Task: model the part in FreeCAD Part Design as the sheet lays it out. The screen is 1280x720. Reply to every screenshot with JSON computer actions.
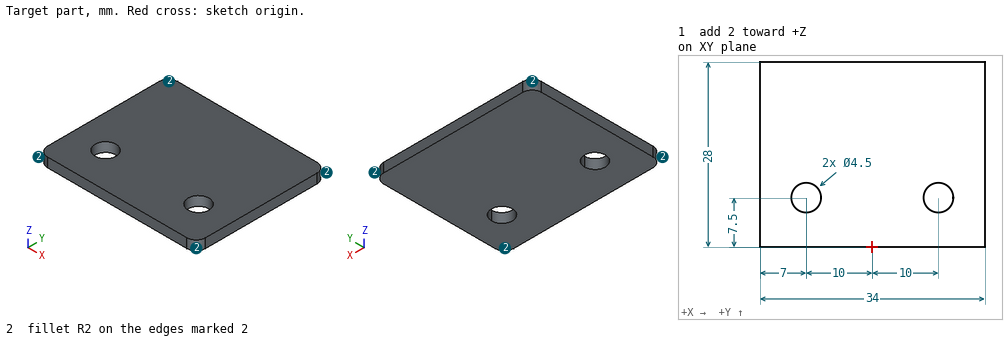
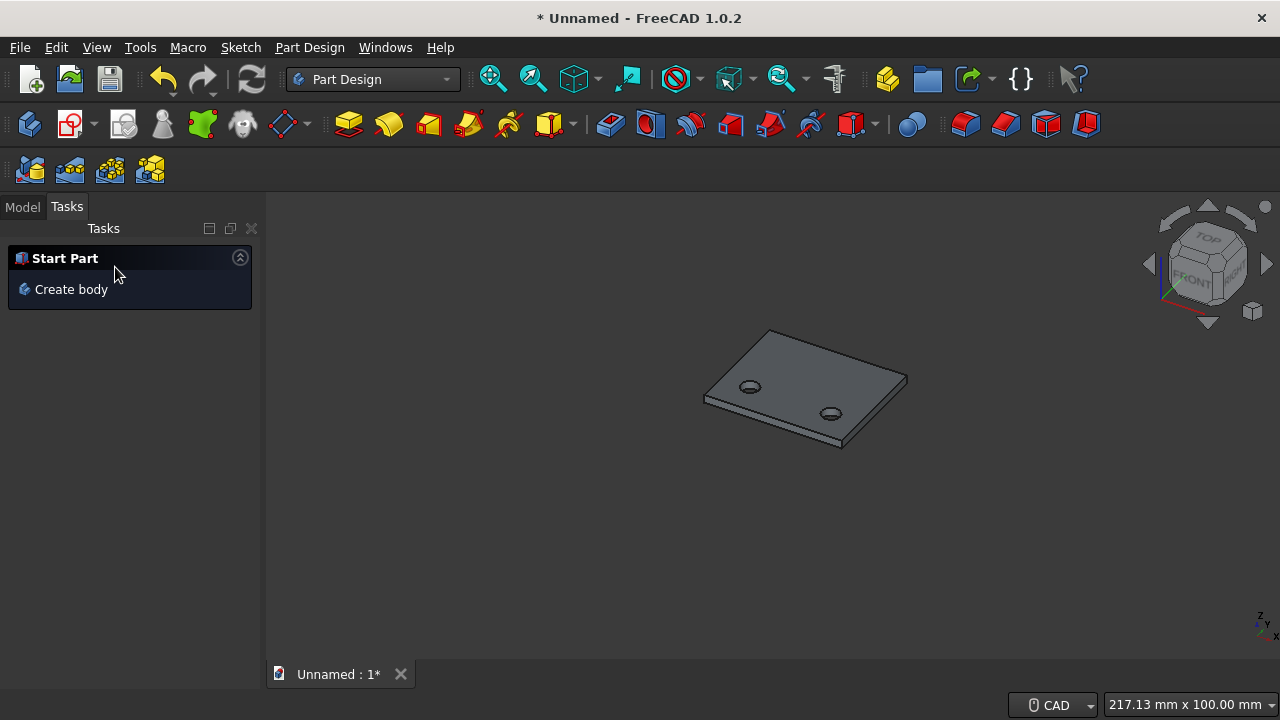
{"action": "key", "text": "v f"}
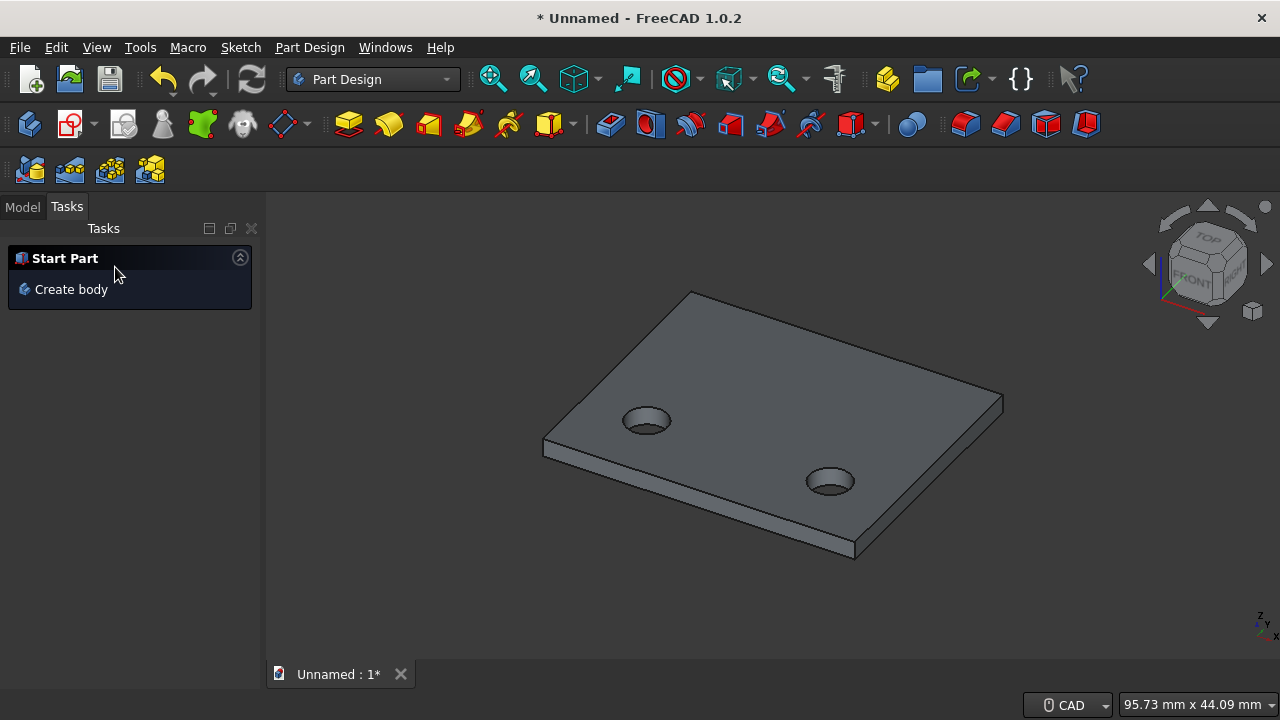
{"action": "left_click", "coordinate": [855, 550]}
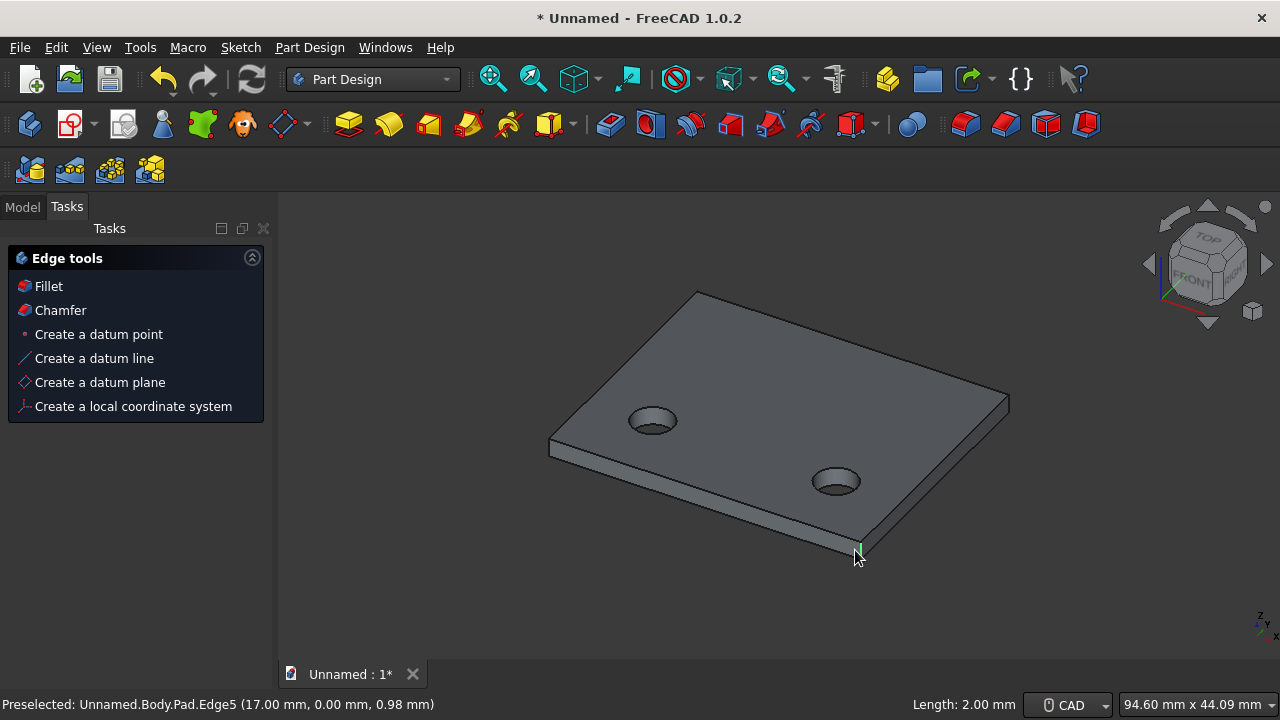
{"action": "scroll", "coordinate": [549, 447], "scroll_direction": "up", "scroll_amount": 4}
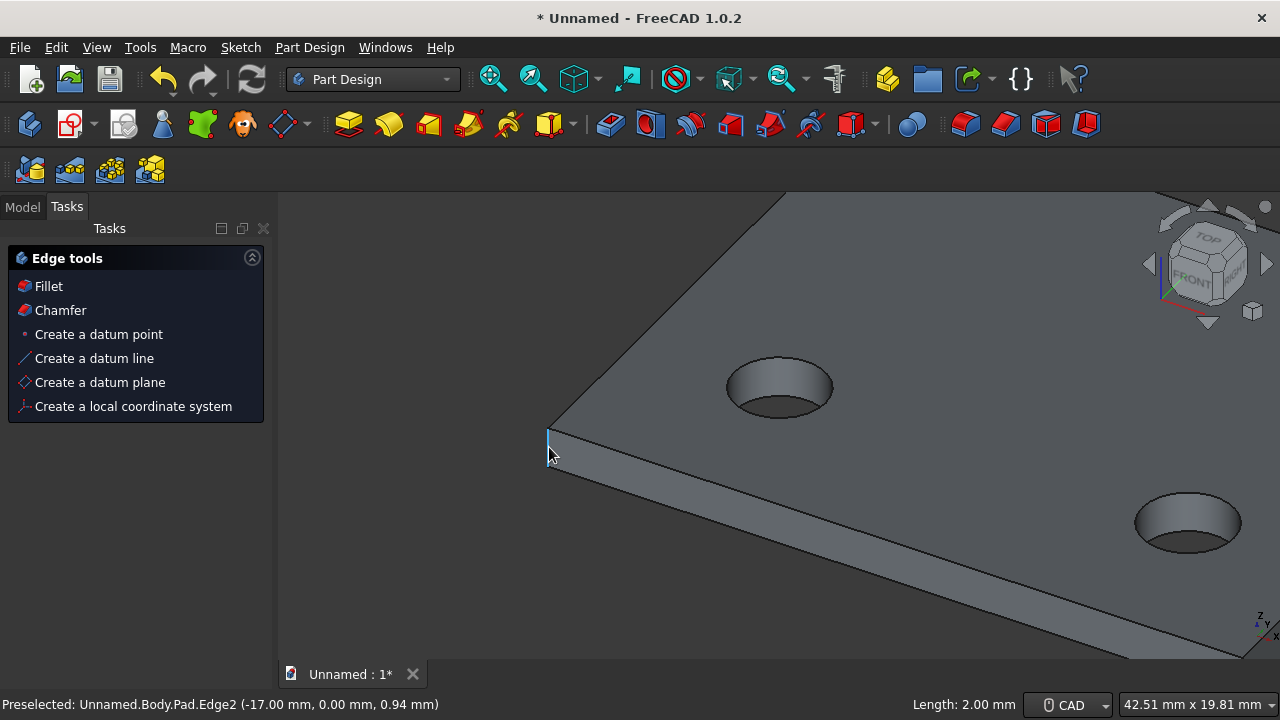
{"action": "key", "text": "v f"}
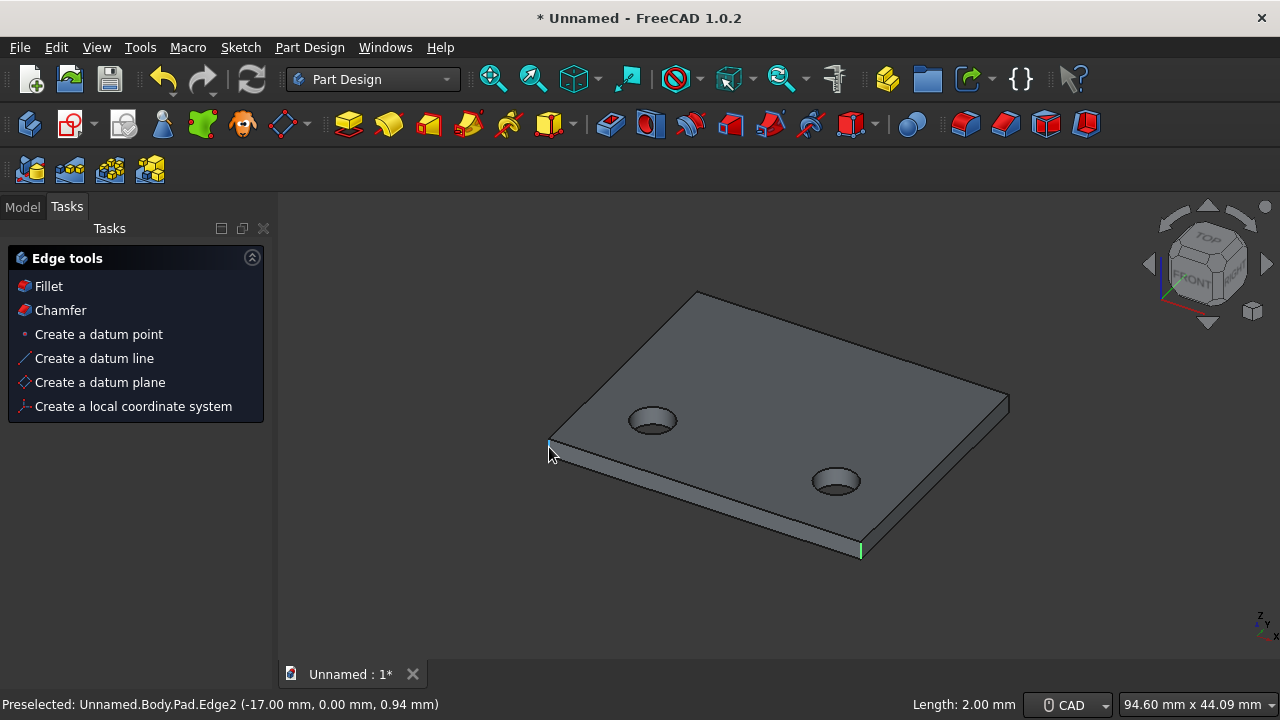
{"action": "key", "text": "0"}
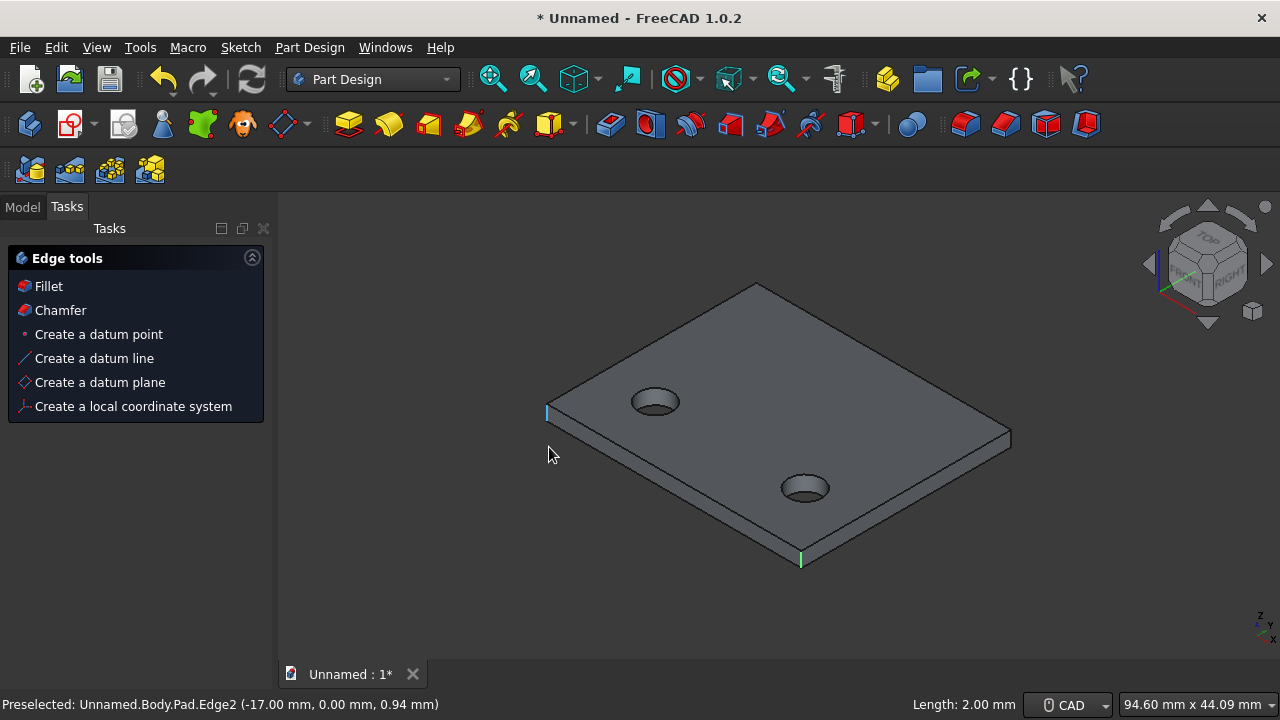
{"action": "scroll", "coordinate": [547, 412], "scroll_direction": "up", "scroll_amount": 4}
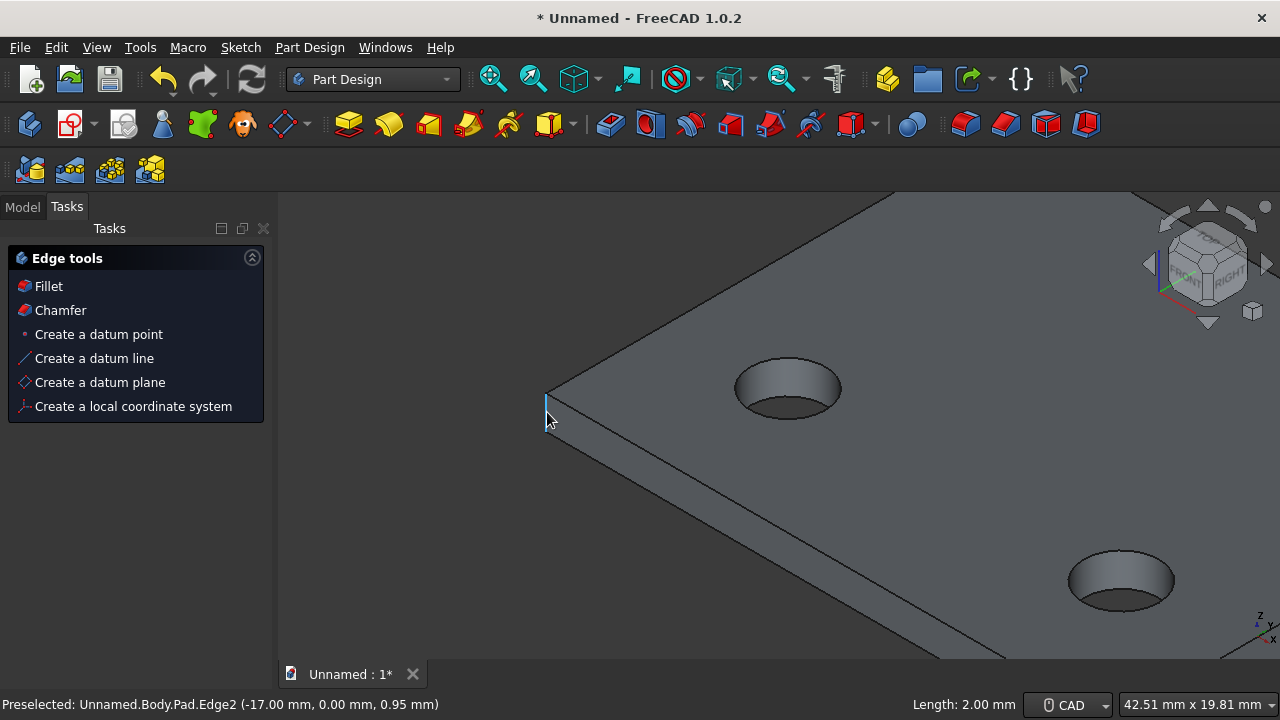
{"action": "key", "text": "v f"}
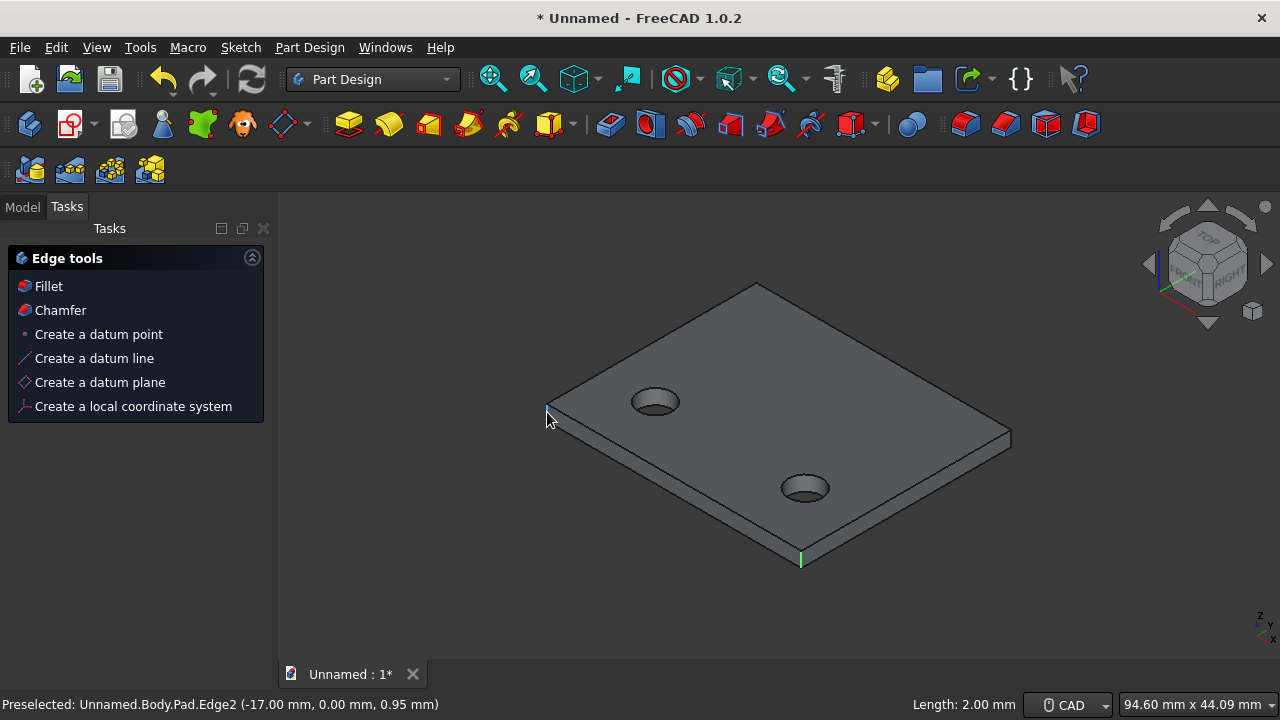
{"action": "key", "text": "2"}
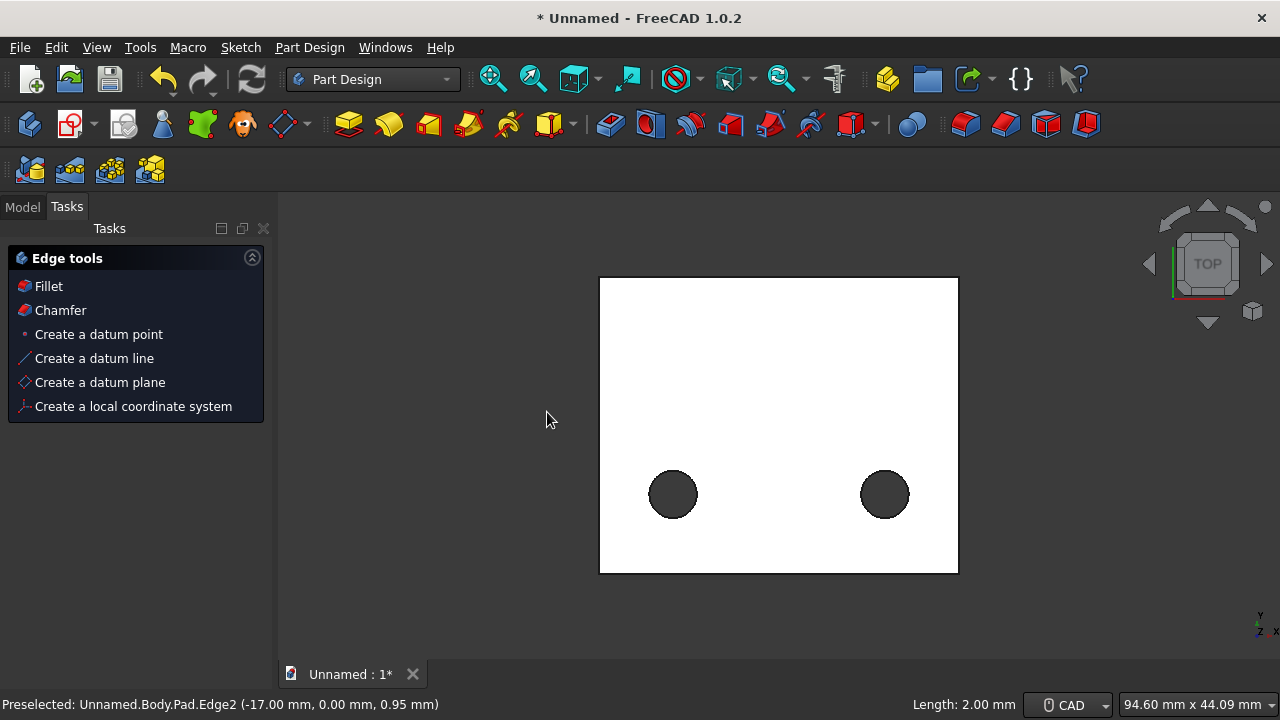
{"action": "scroll", "coordinate": [599, 573], "scroll_direction": "up", "scroll_amount": 4}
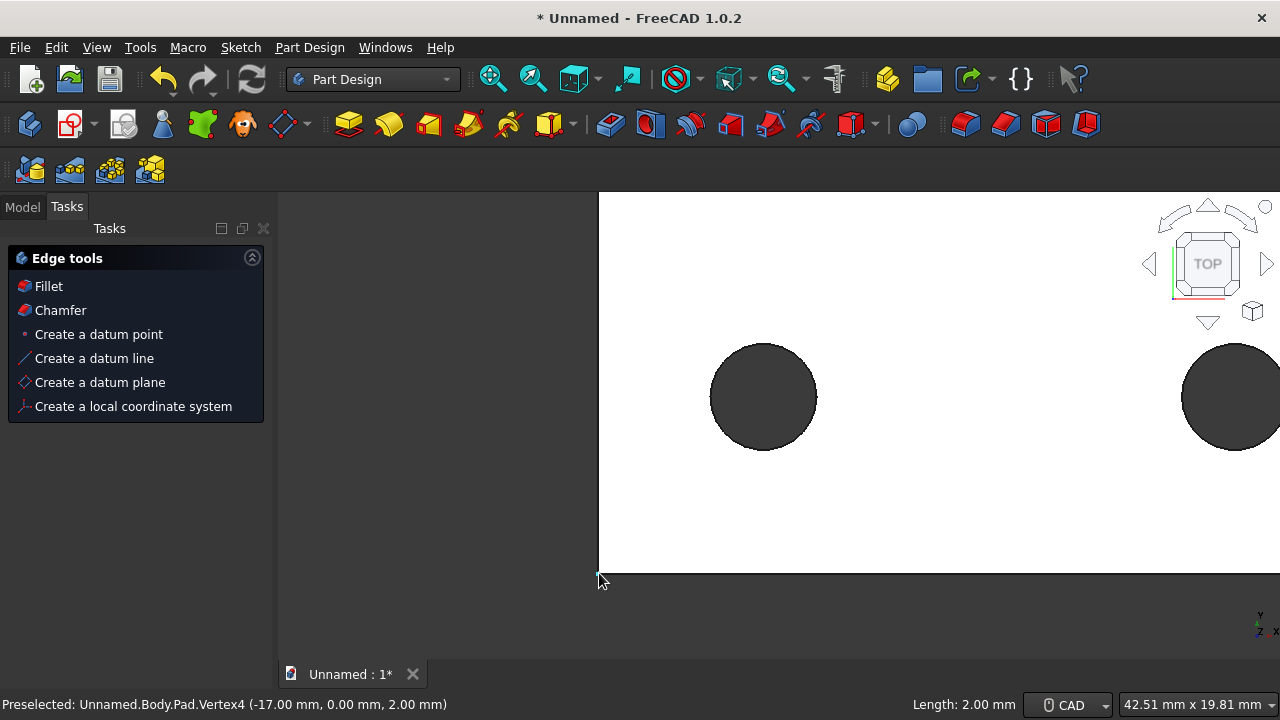
{"action": "key", "text": "v f"}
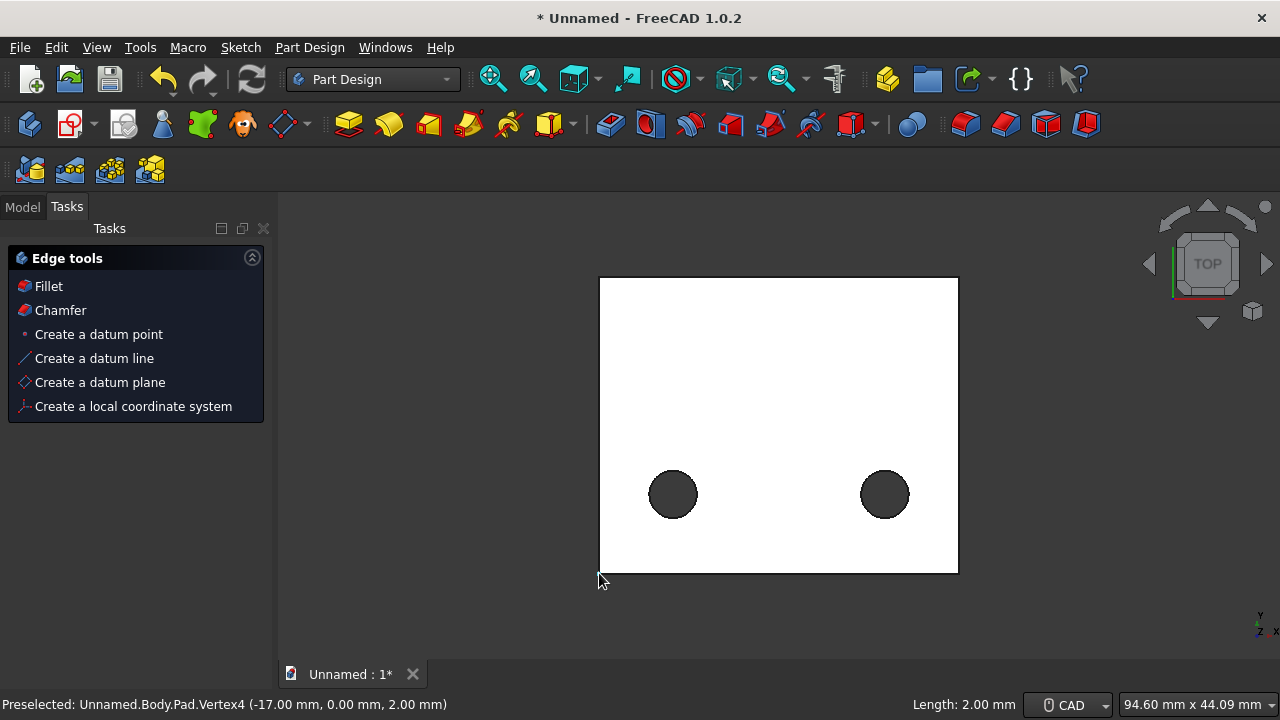
{"action": "key", "text": "1"}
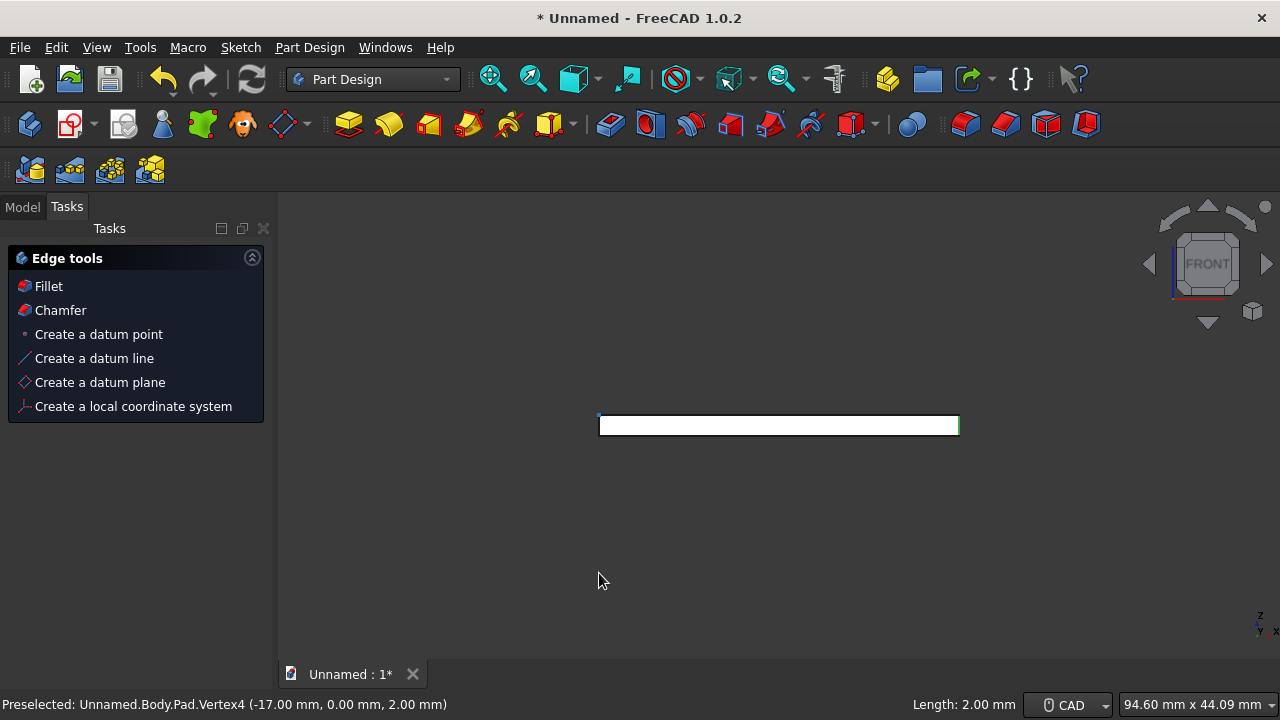
{"action": "key", "text": "v f"}